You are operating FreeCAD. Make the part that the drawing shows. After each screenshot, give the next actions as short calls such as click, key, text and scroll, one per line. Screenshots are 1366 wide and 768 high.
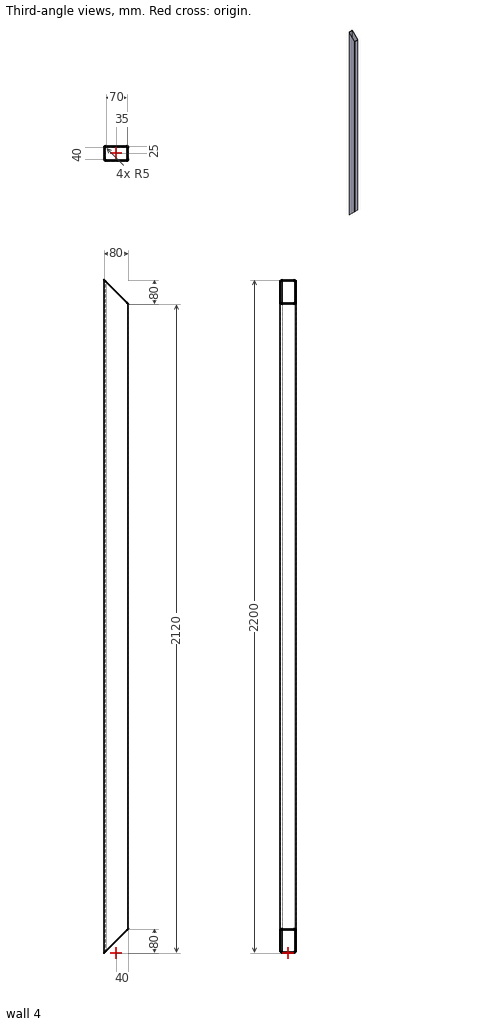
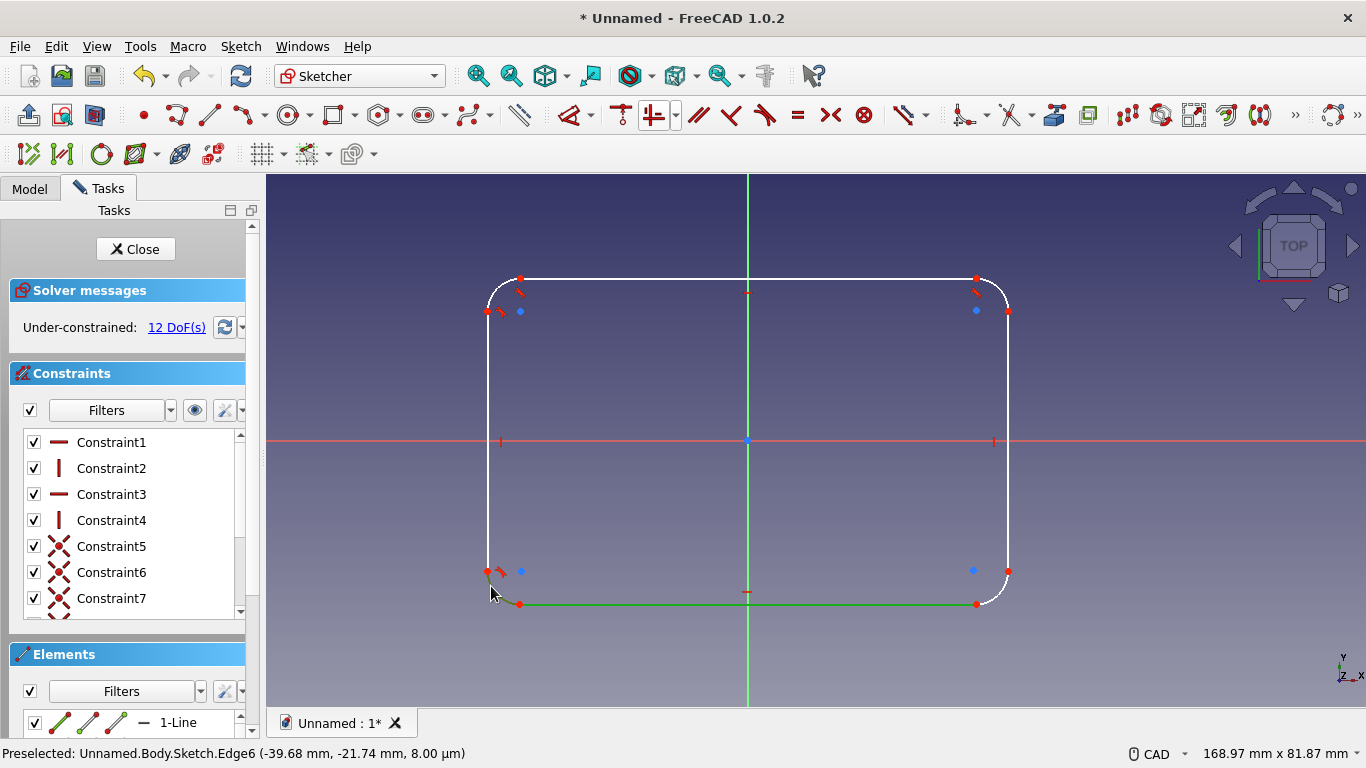
click(765, 116)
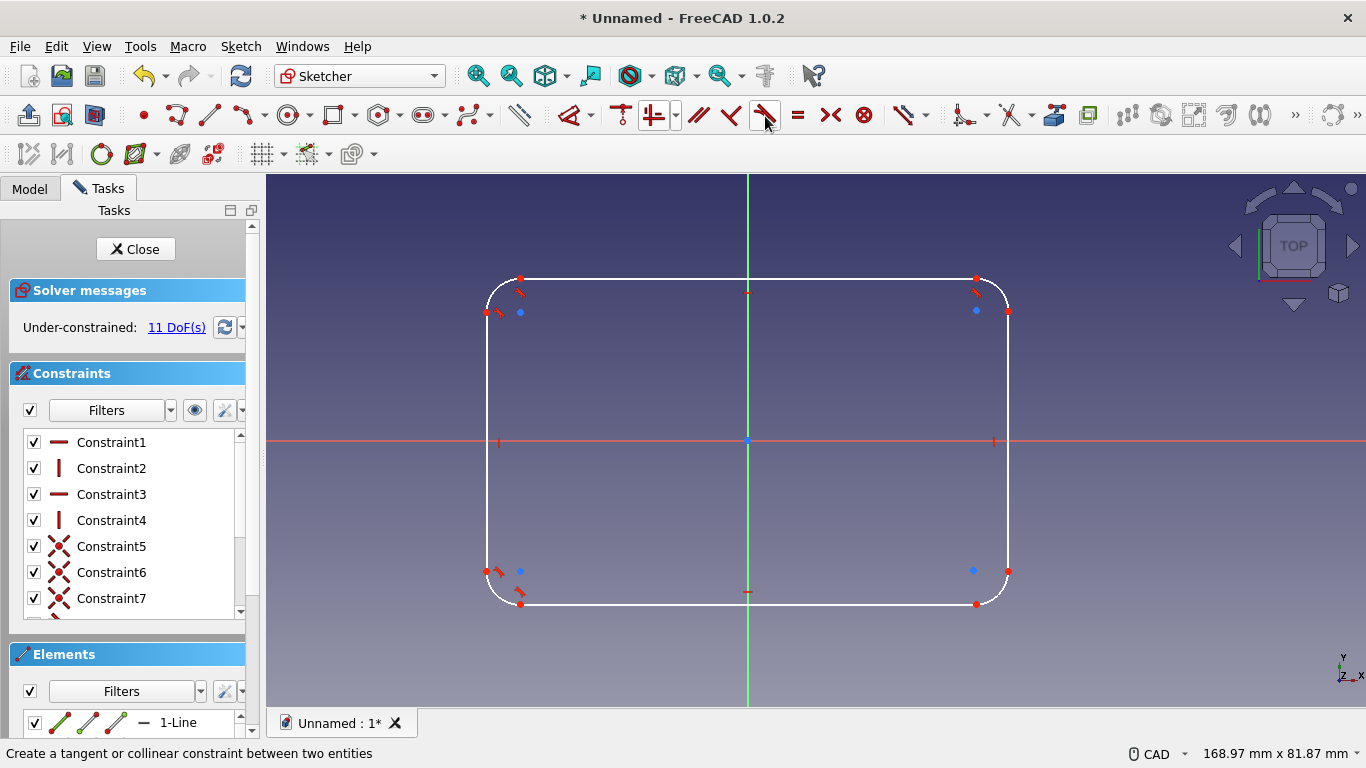
click(657, 605)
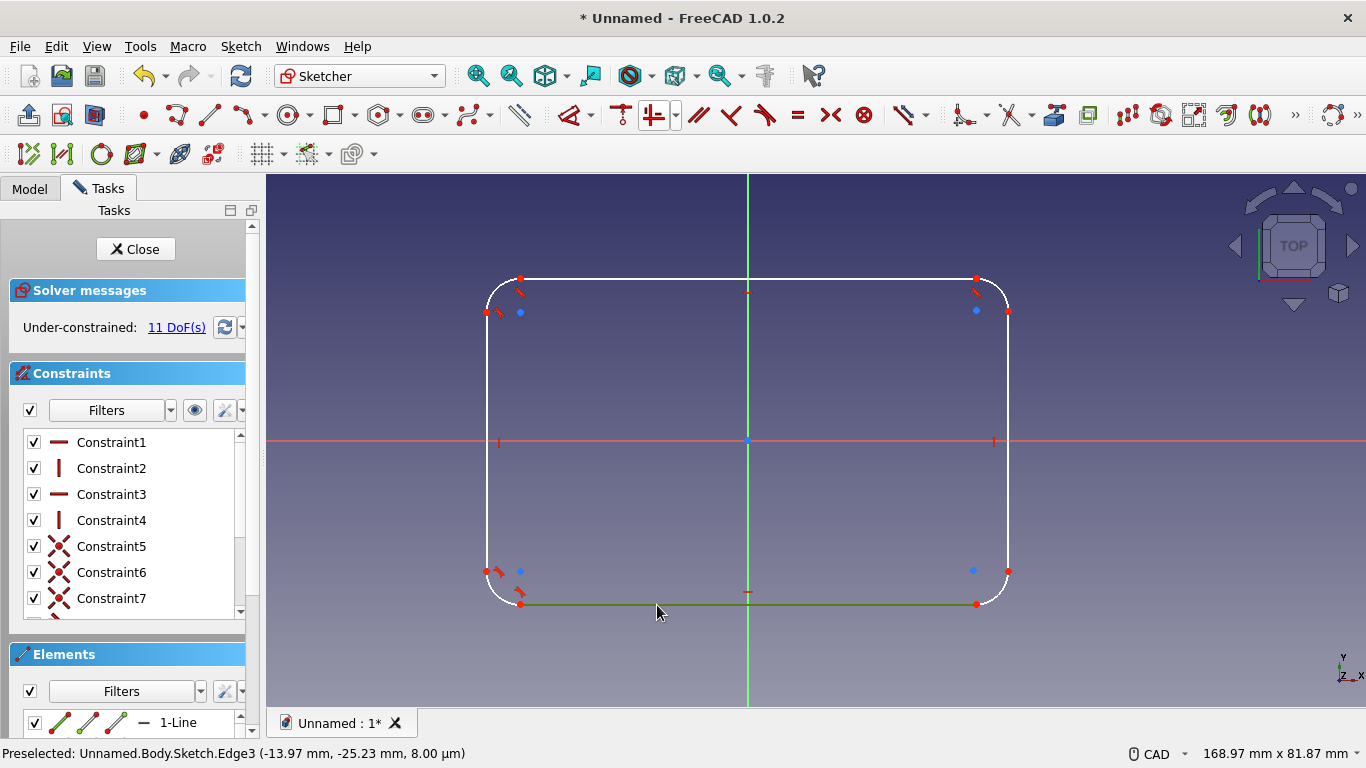
click(991, 601)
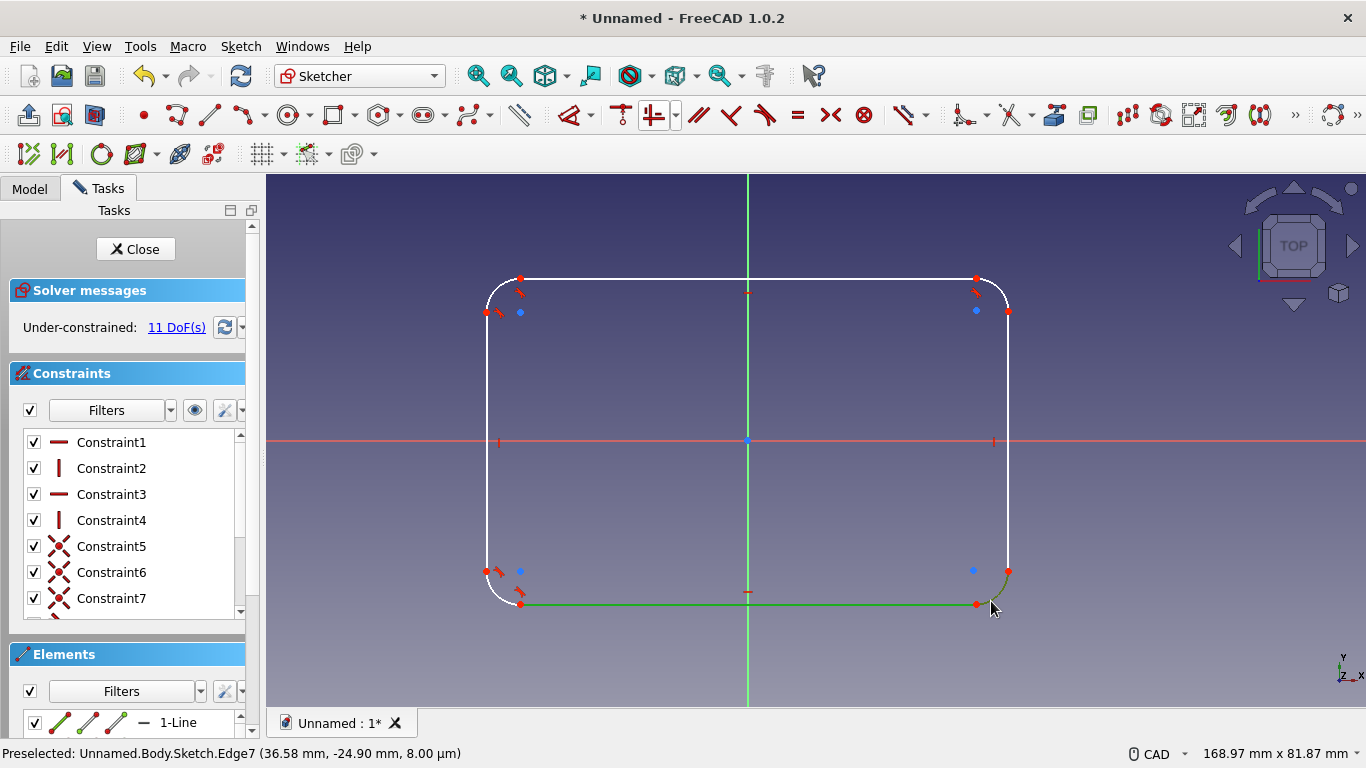
click(765, 116)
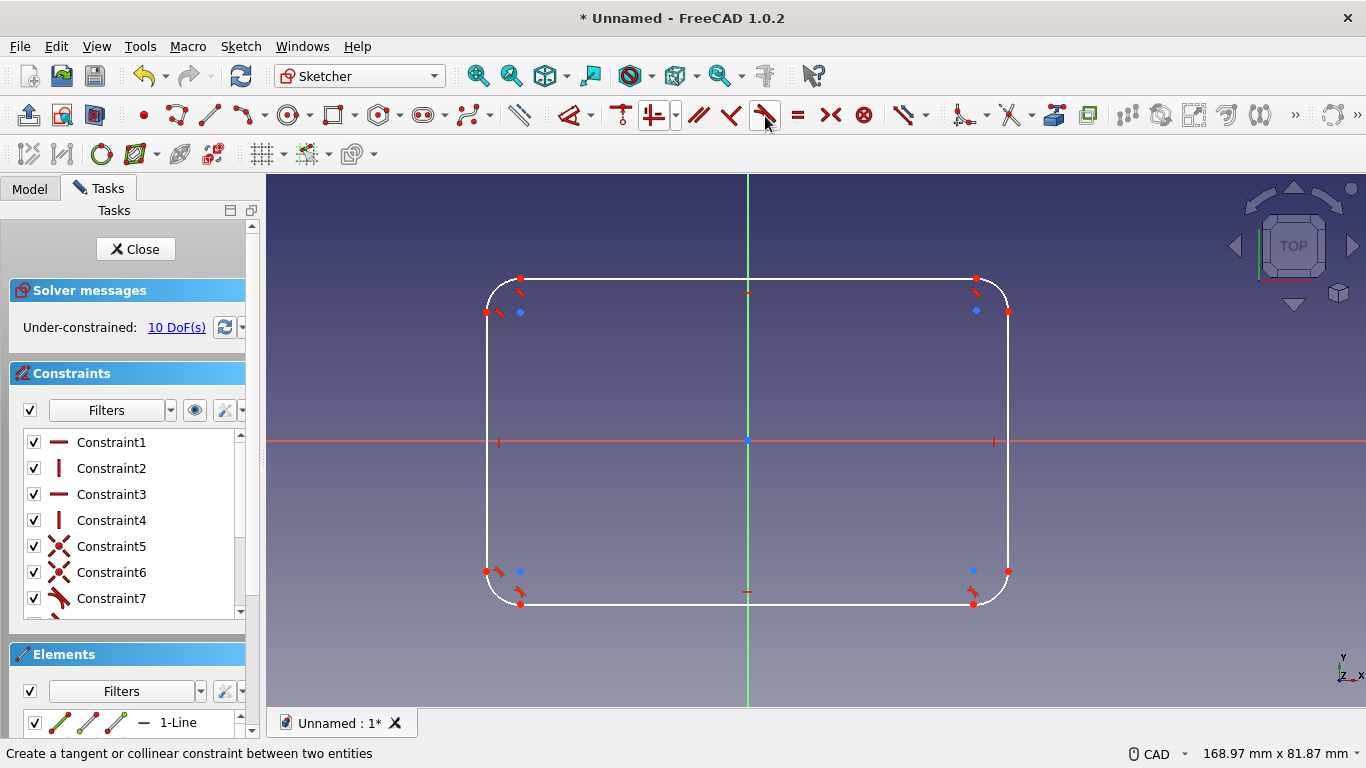
click(1008, 494)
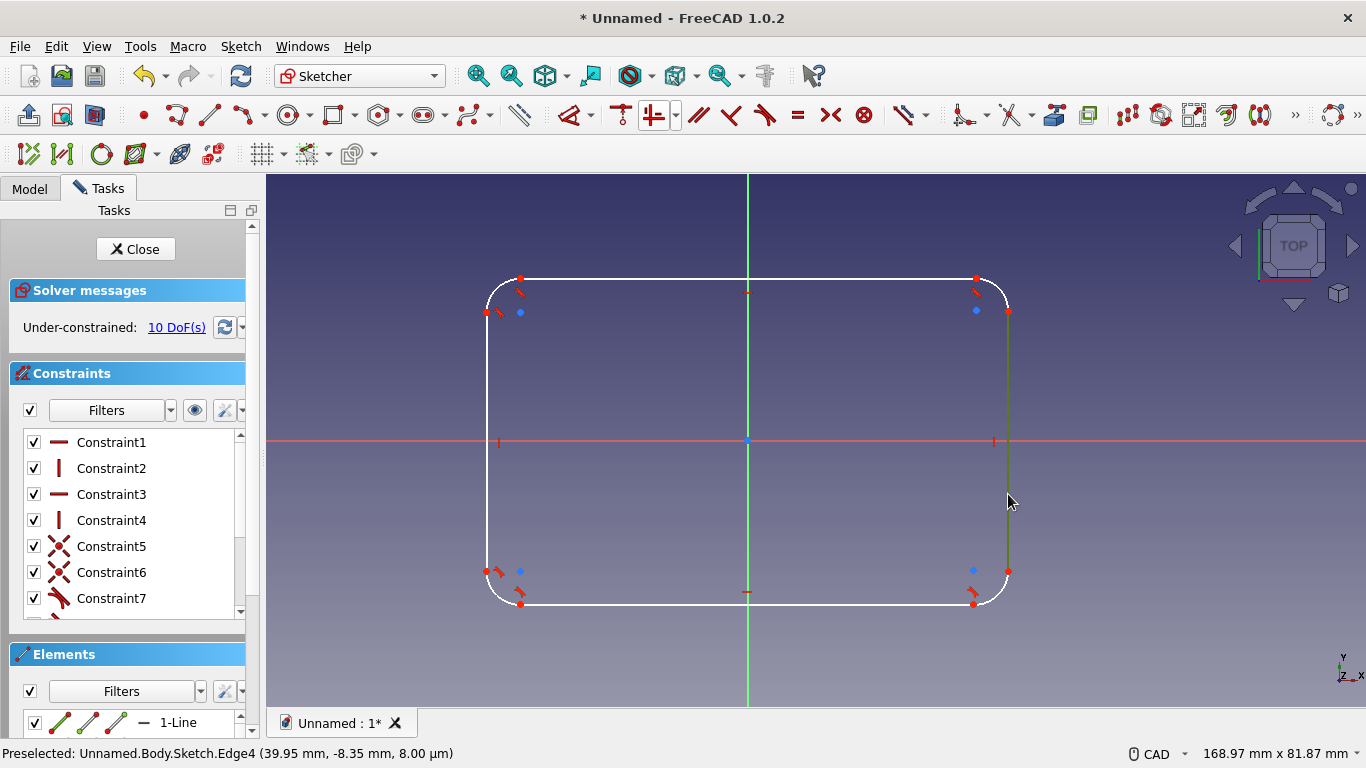
click(989, 601)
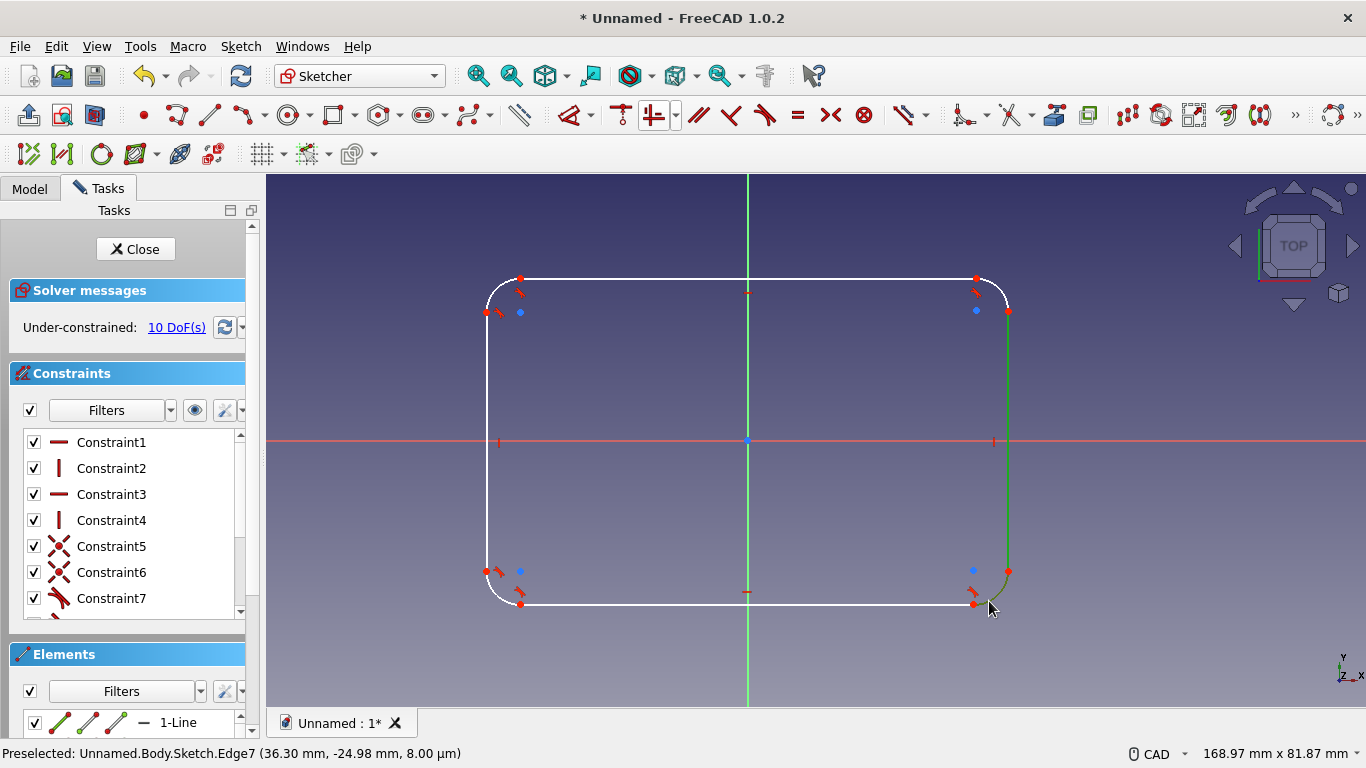
click(765, 116)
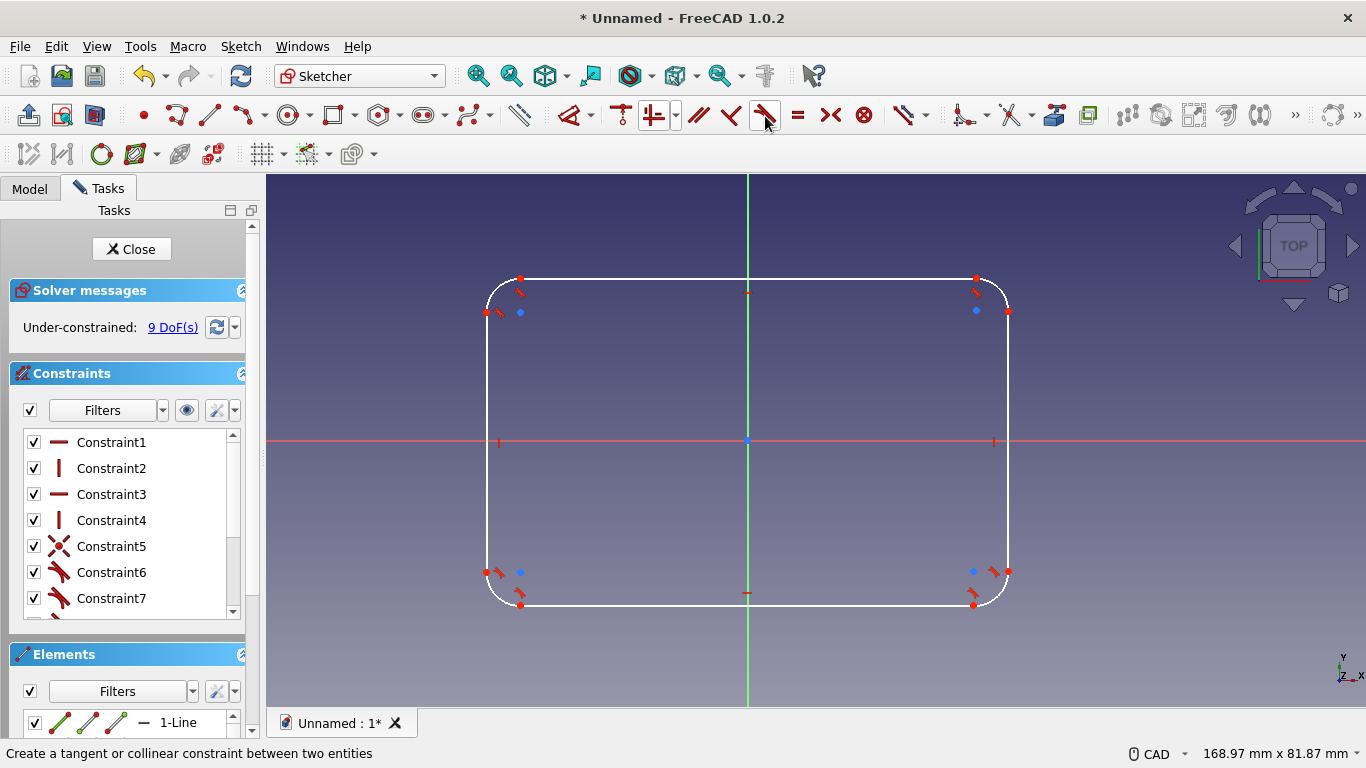
click(1008, 494)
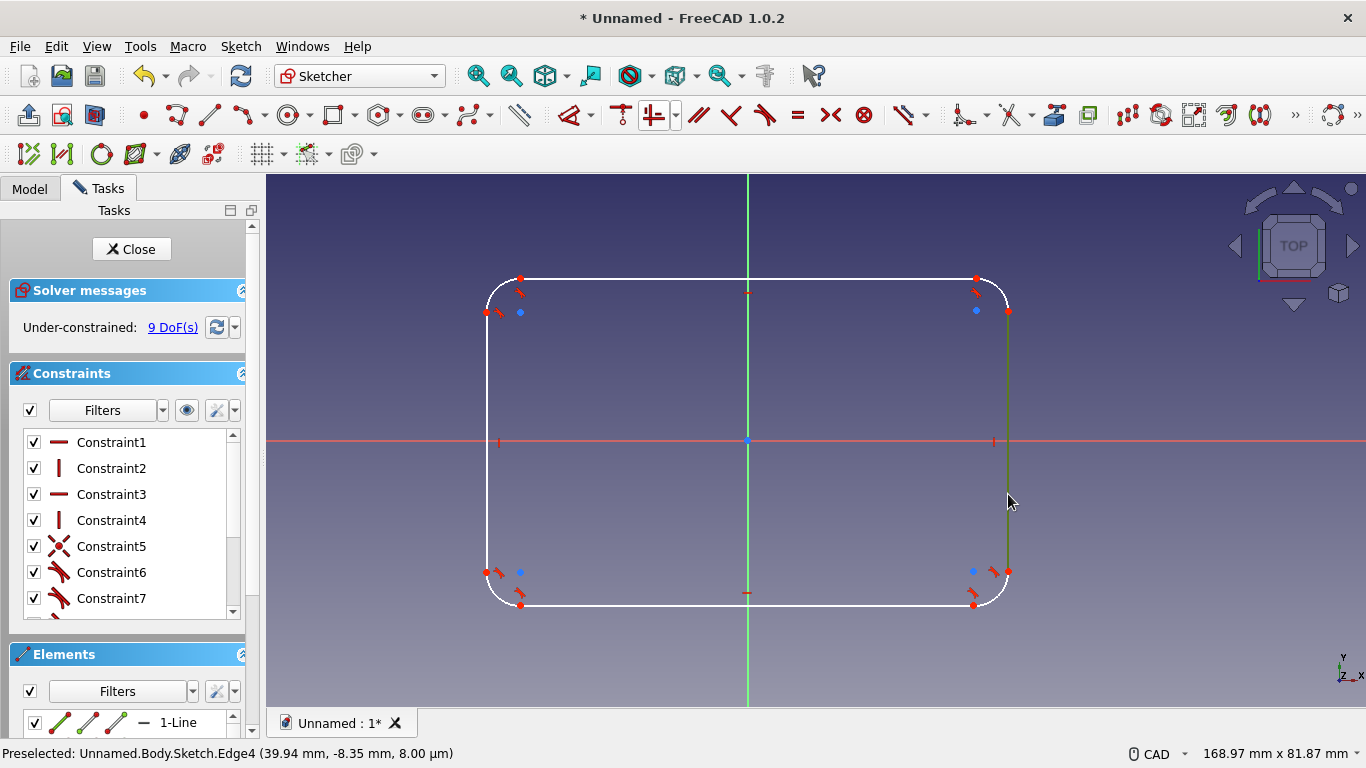
click(1005, 297)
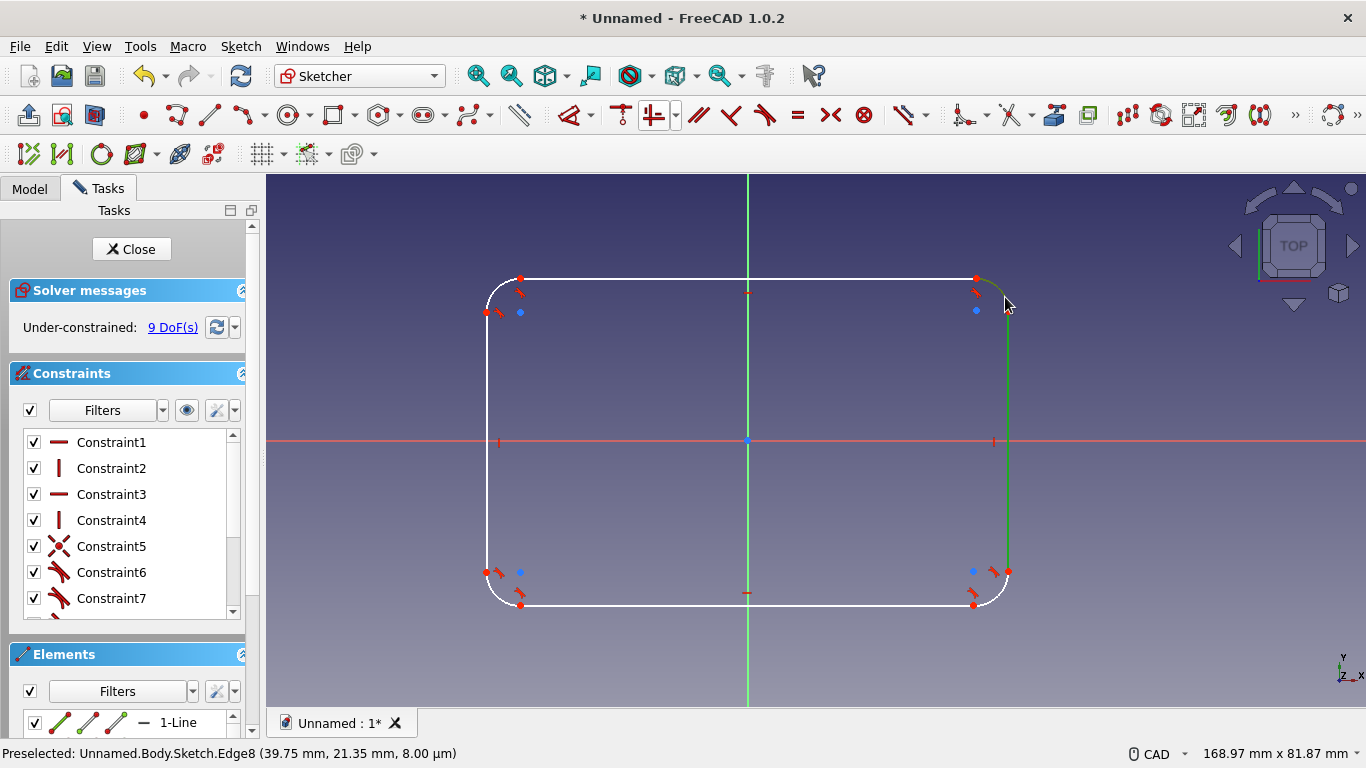
click(765, 116)